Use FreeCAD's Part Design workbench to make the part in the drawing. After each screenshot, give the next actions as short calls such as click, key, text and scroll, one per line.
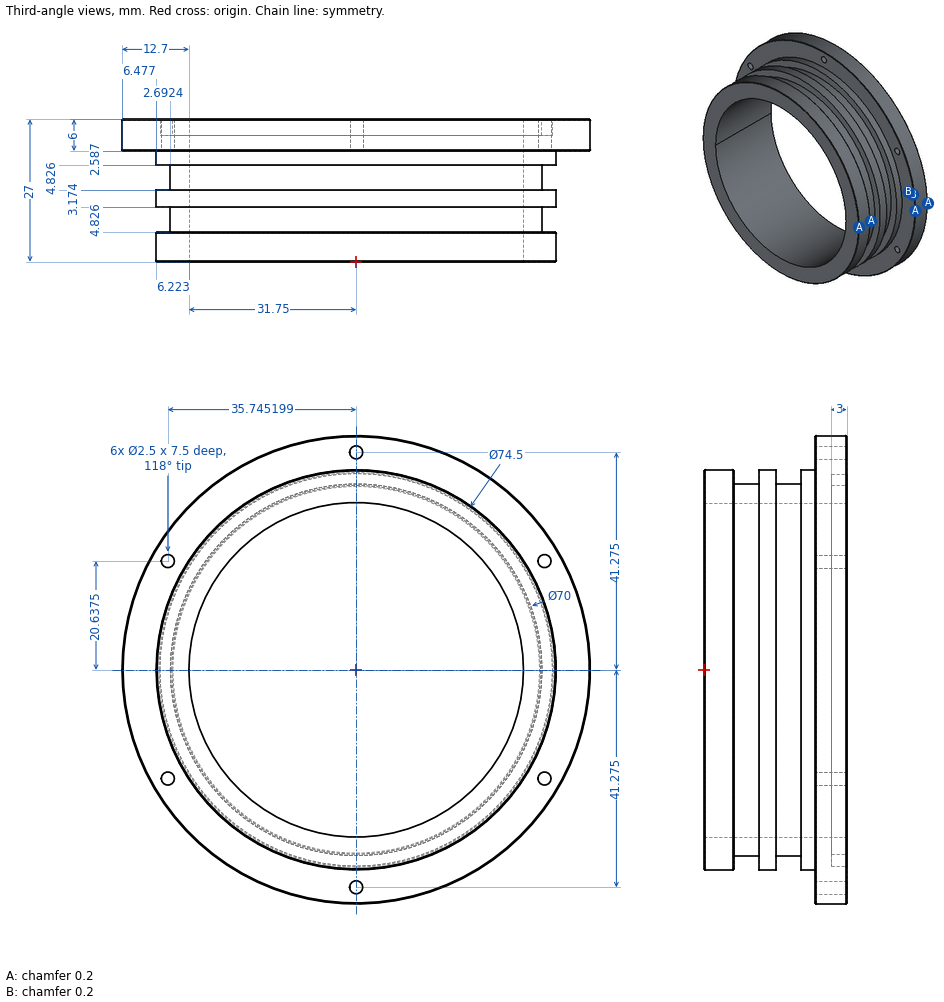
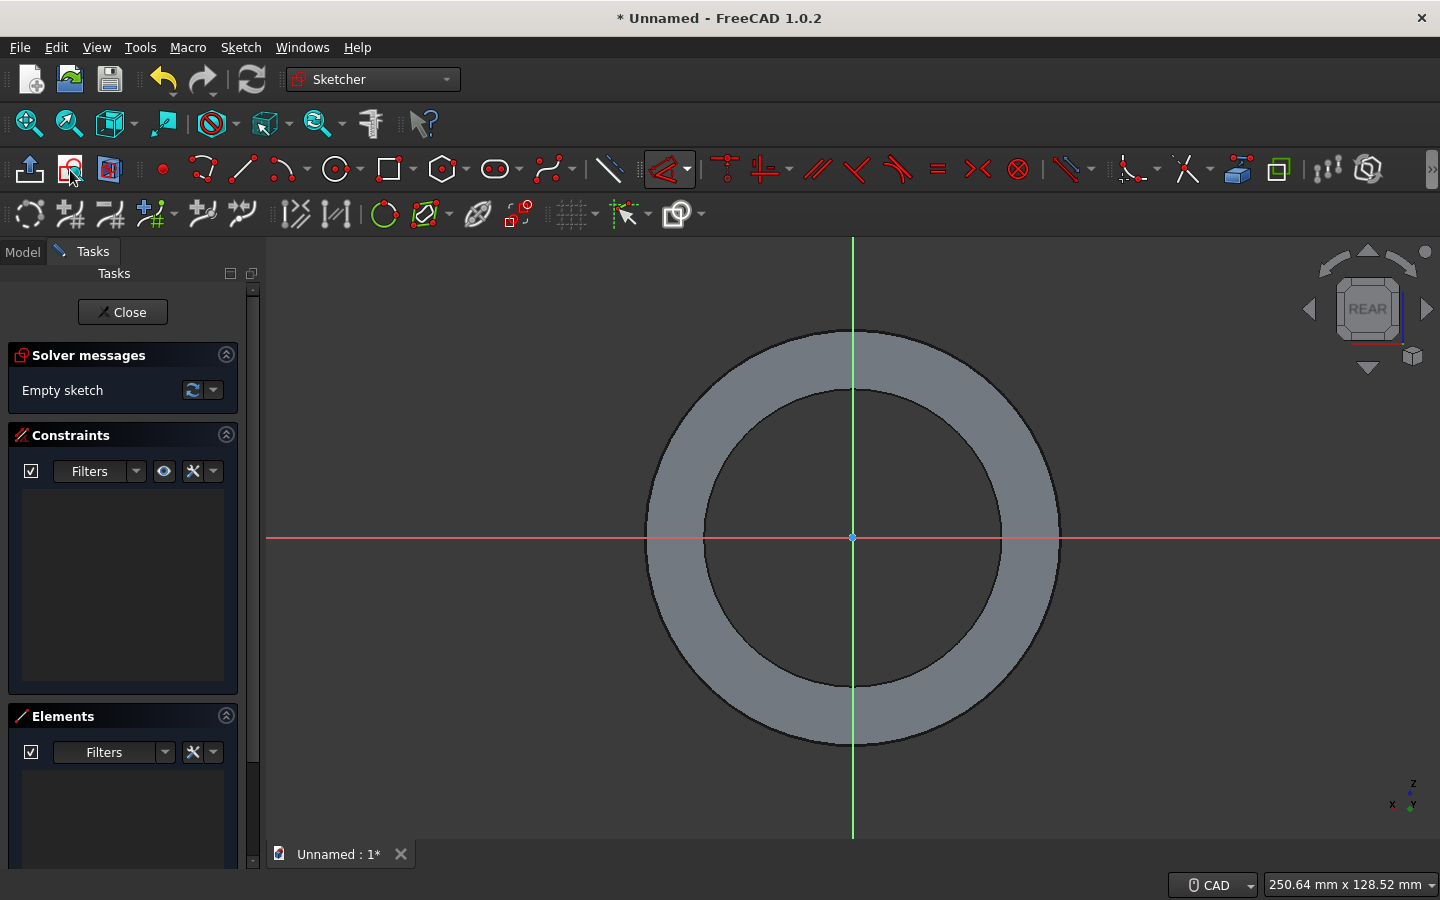
click(336, 170)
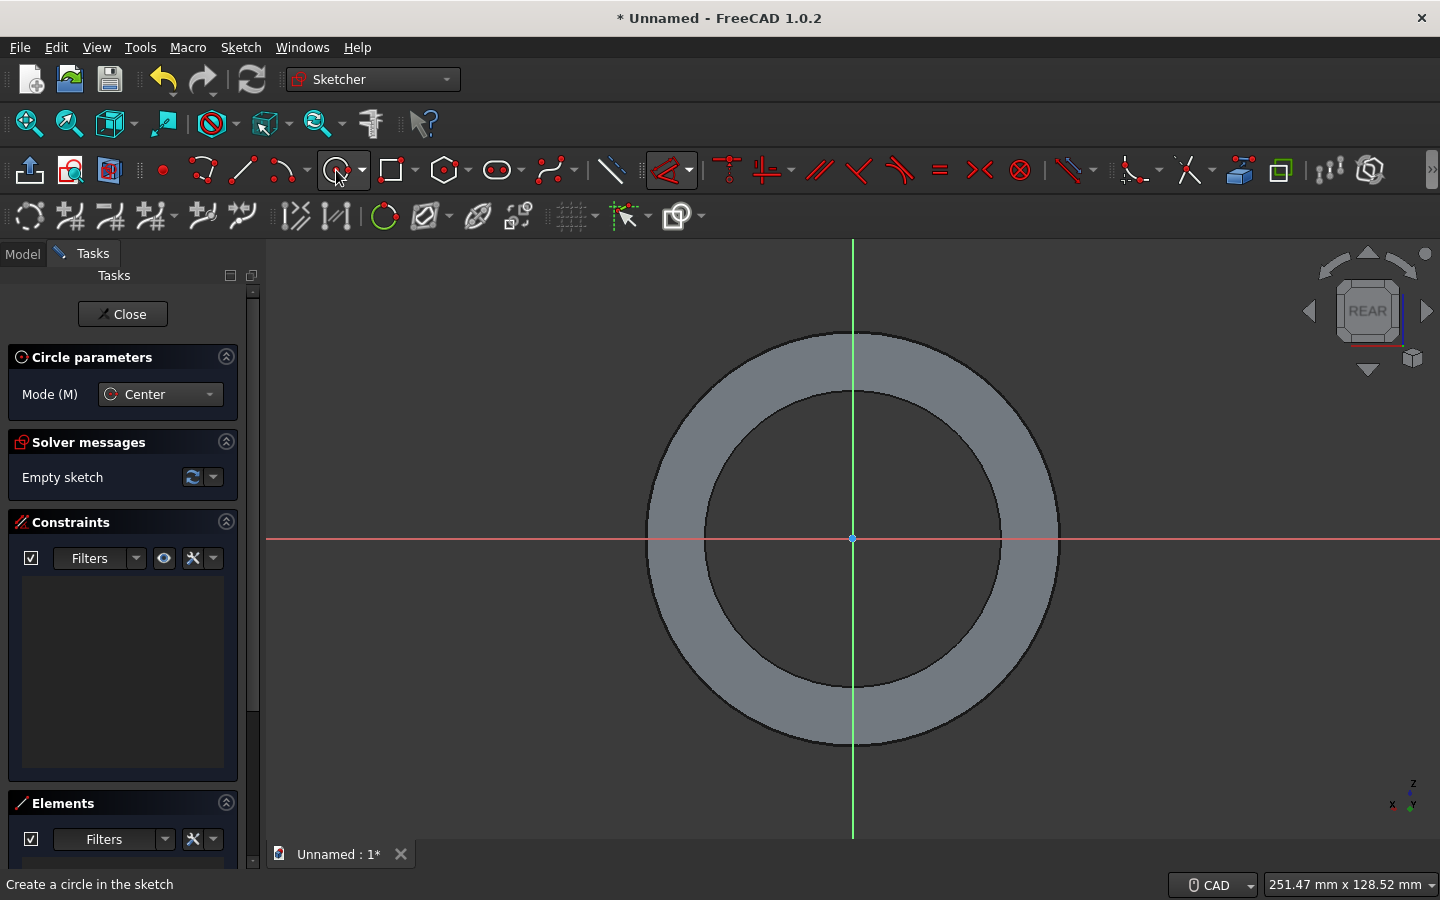
scroll(1020, 443, up, 7)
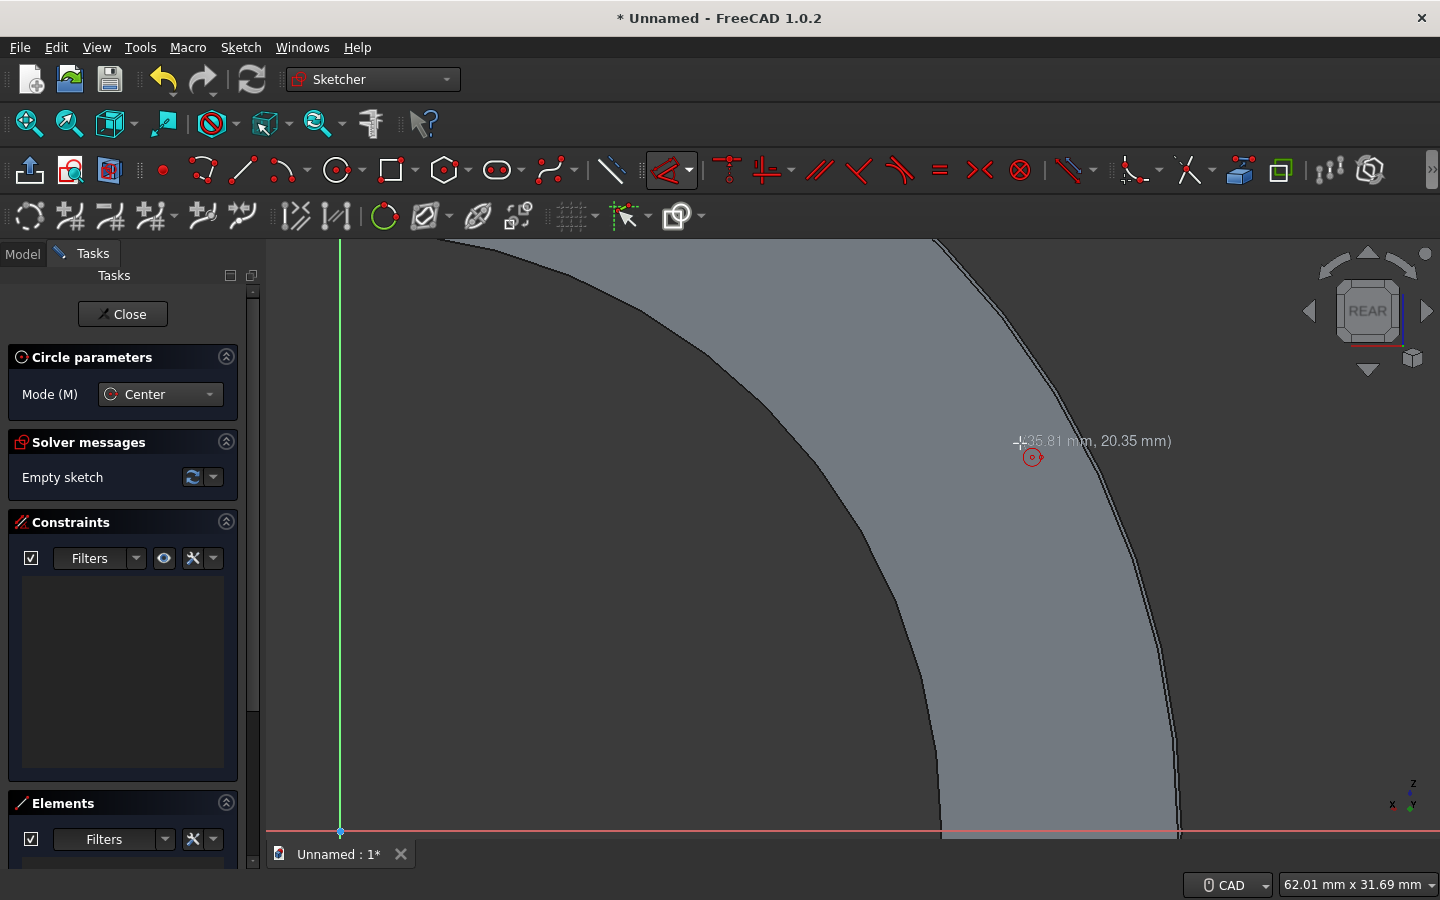
scroll(930, 443, down, 7)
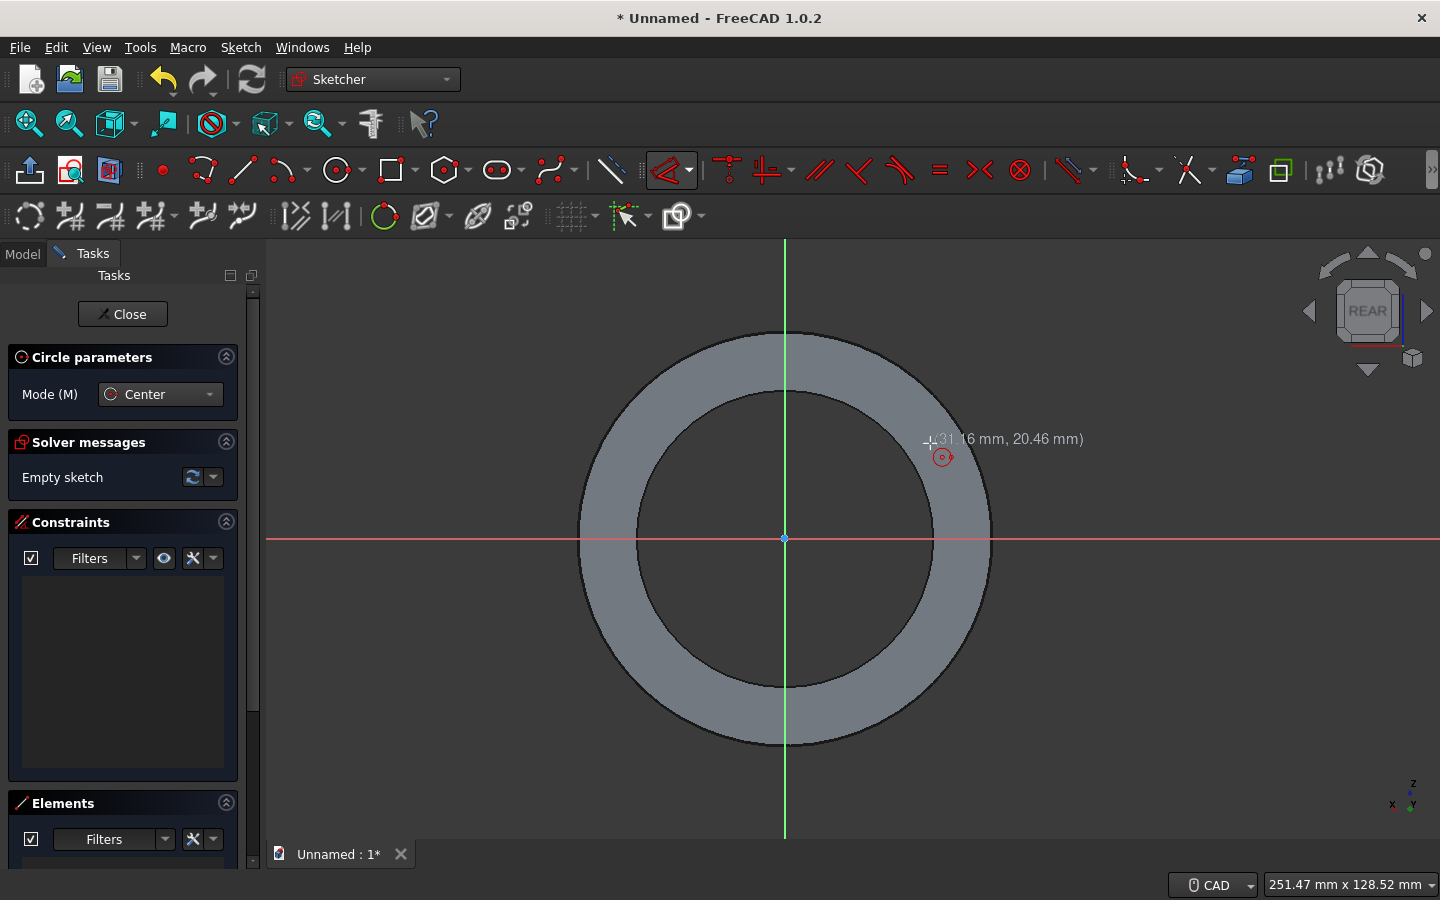
click(952, 443)
move(956, 439)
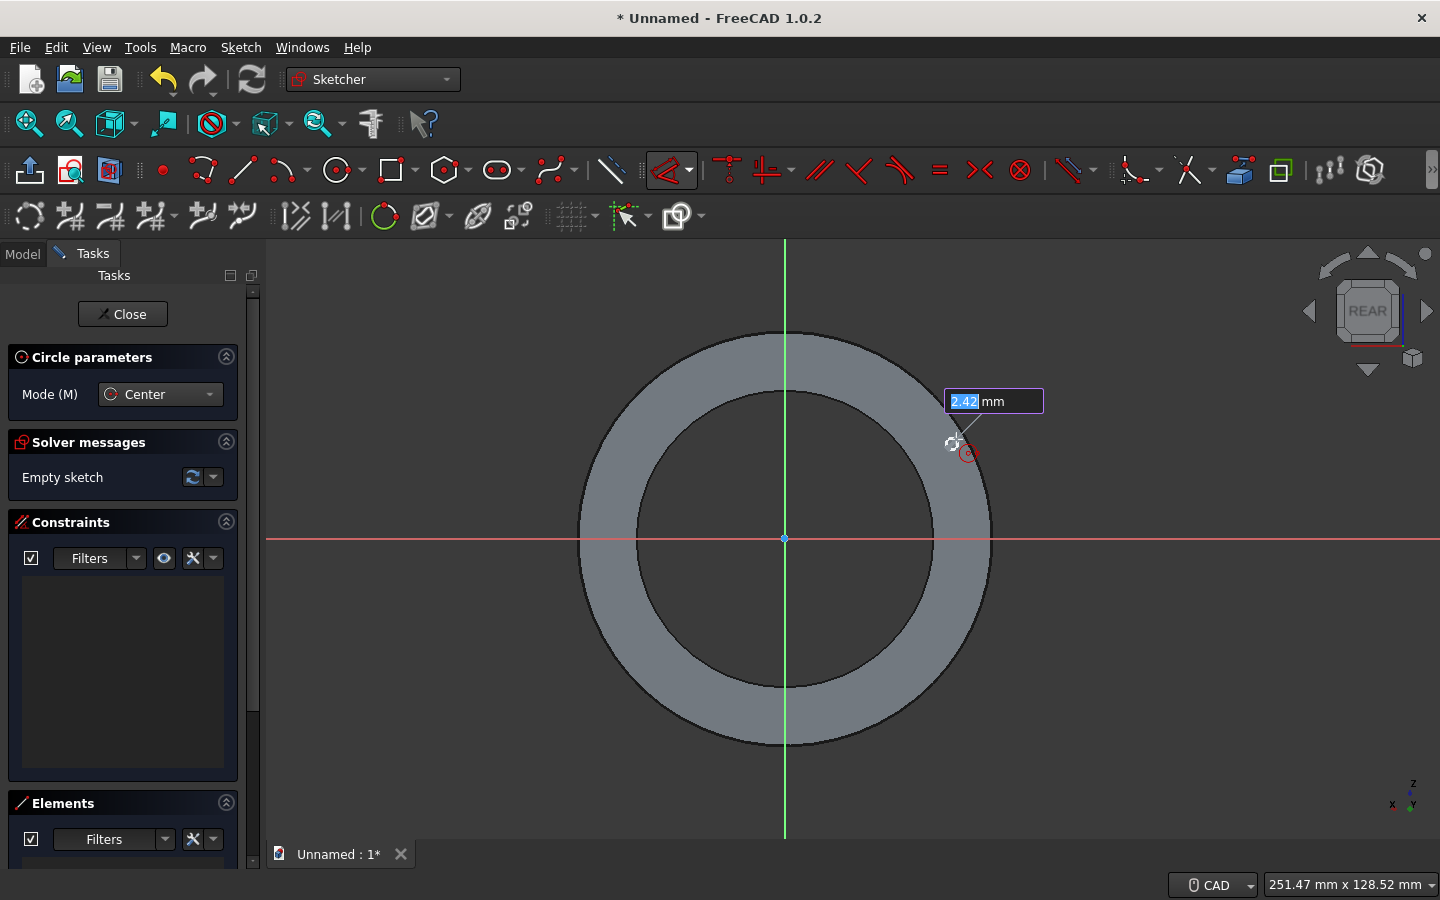
text(2.5)
key(Return)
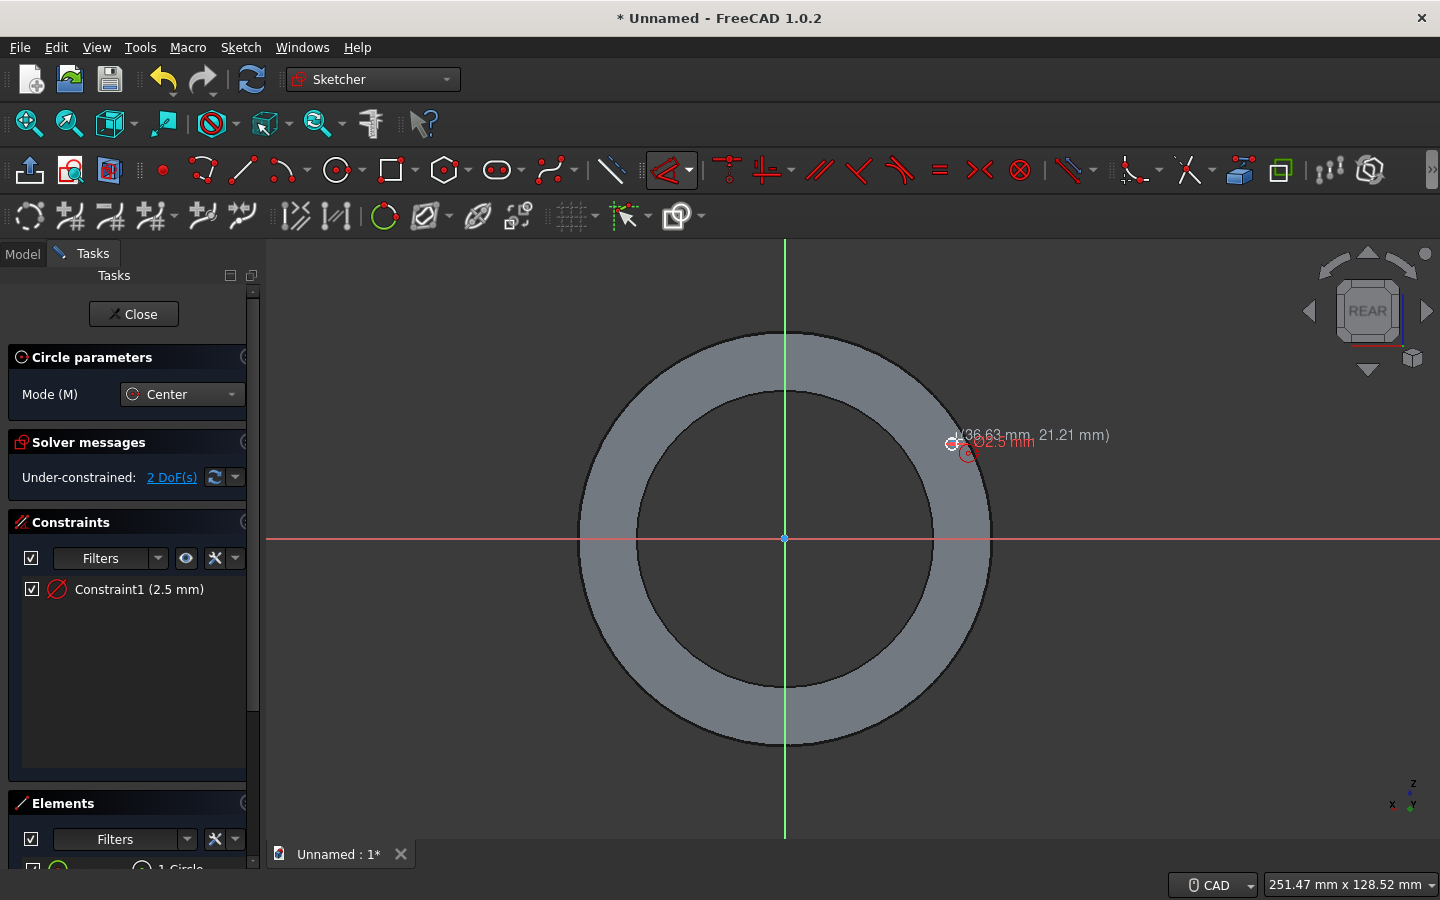
scroll(952, 635, up, 7)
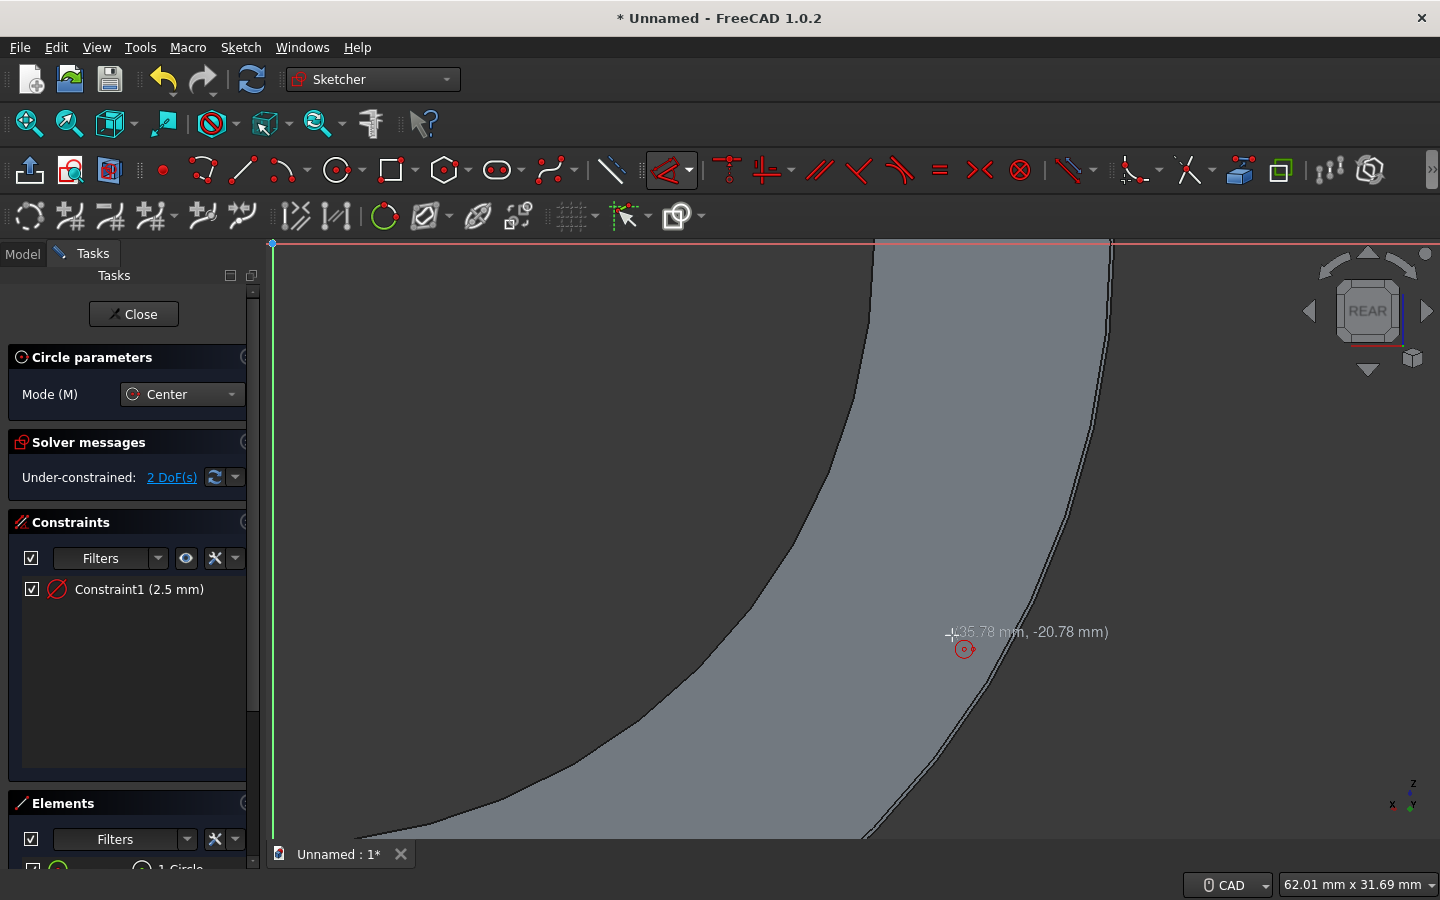
scroll(952, 636, down, 7)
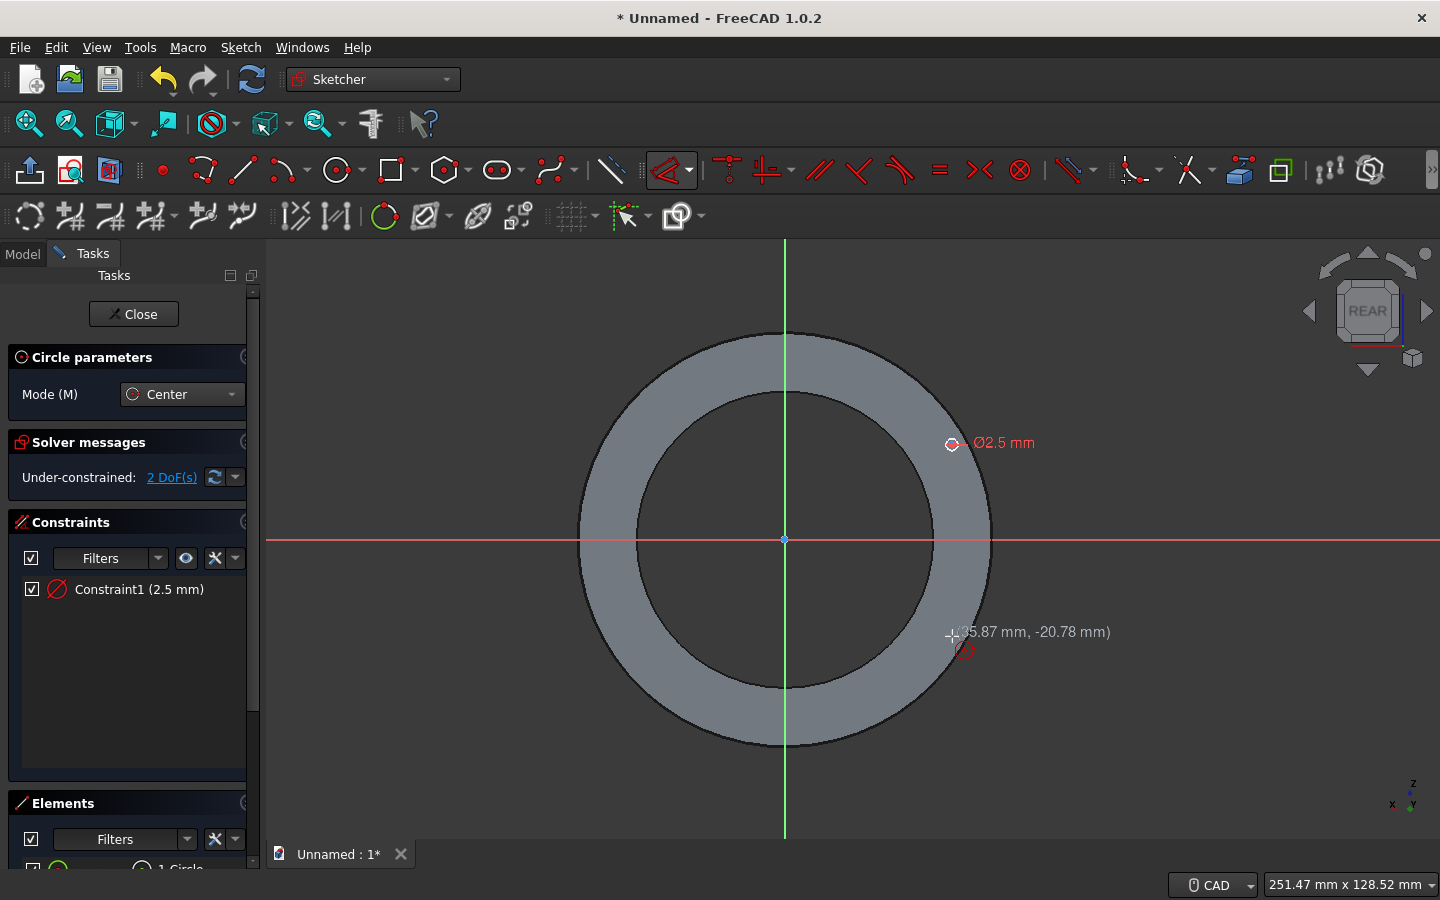
click(952, 636)
move(956, 632)